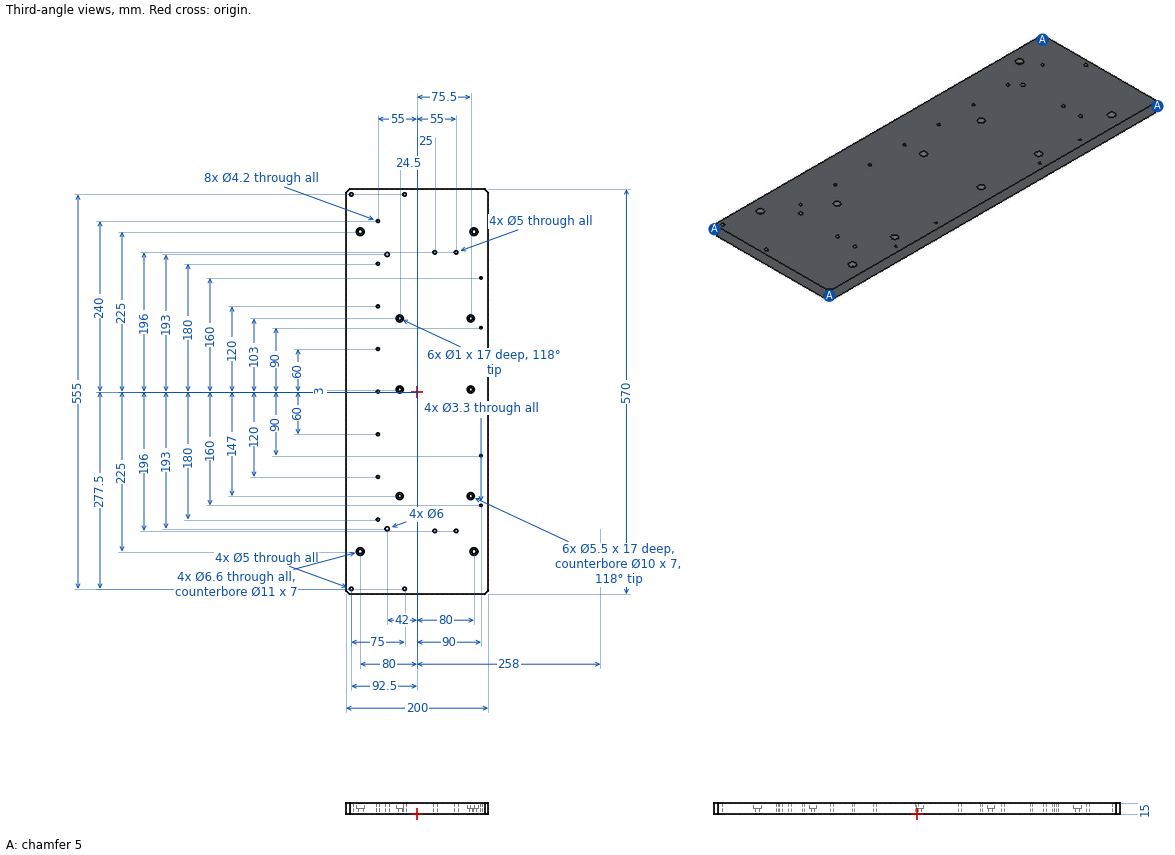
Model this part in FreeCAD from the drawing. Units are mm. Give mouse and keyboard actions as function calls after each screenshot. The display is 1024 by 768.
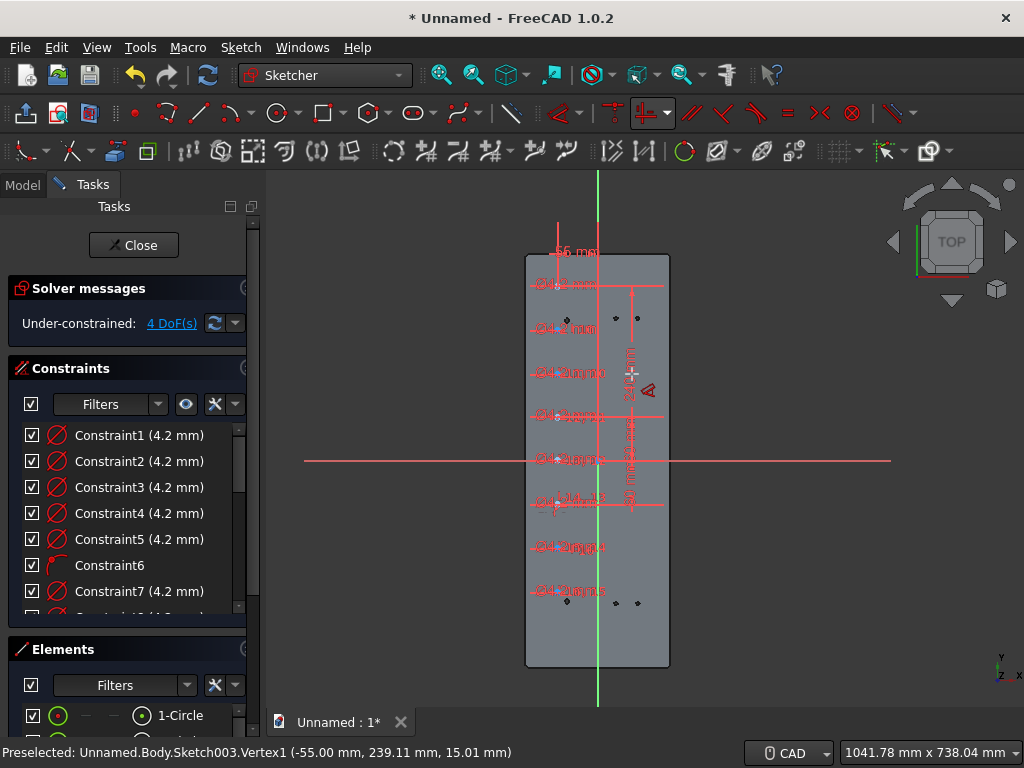
click(558, 331)
click(632, 396)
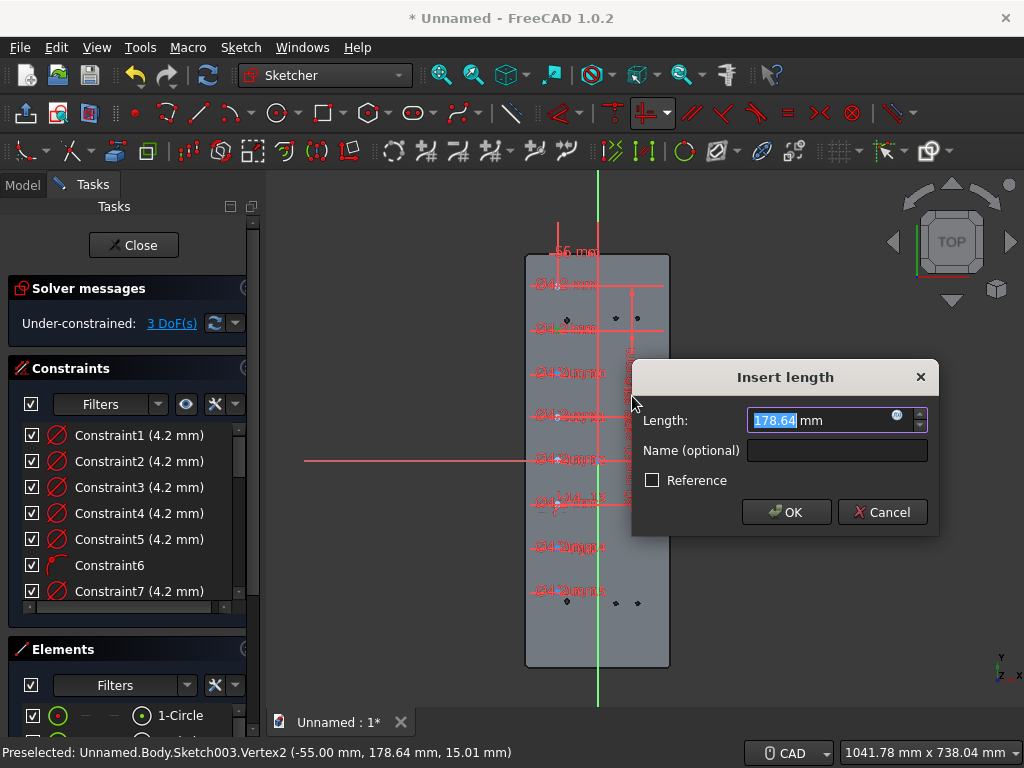
text(180)
key(Return)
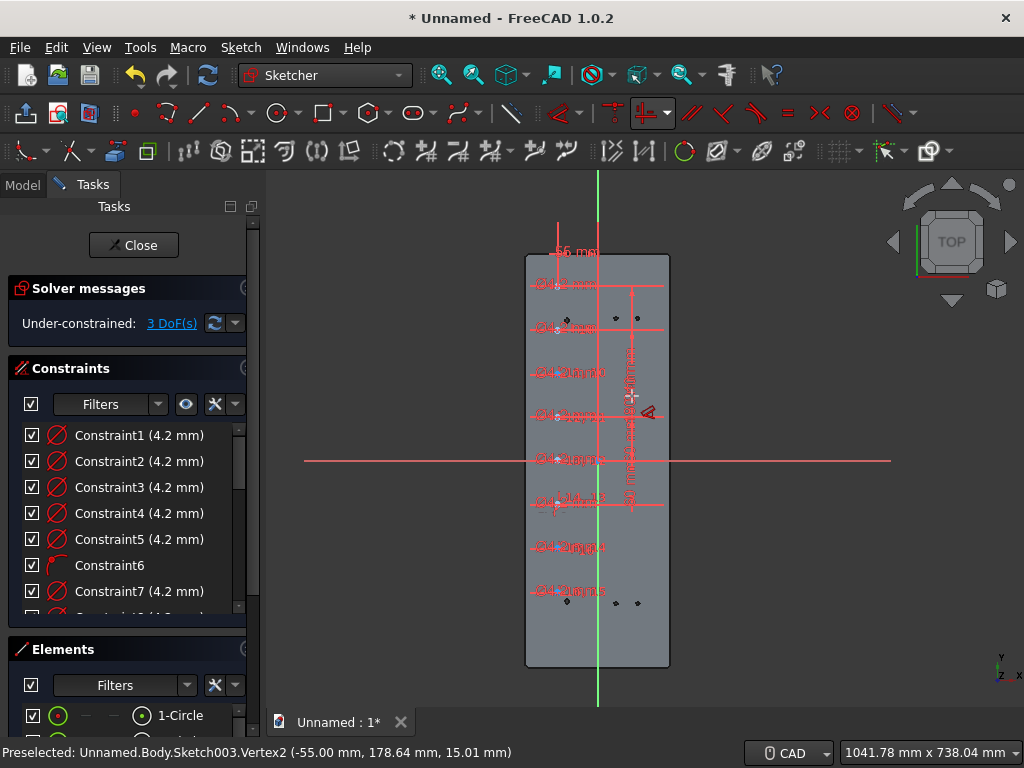
click(558, 375)
click(632, 418)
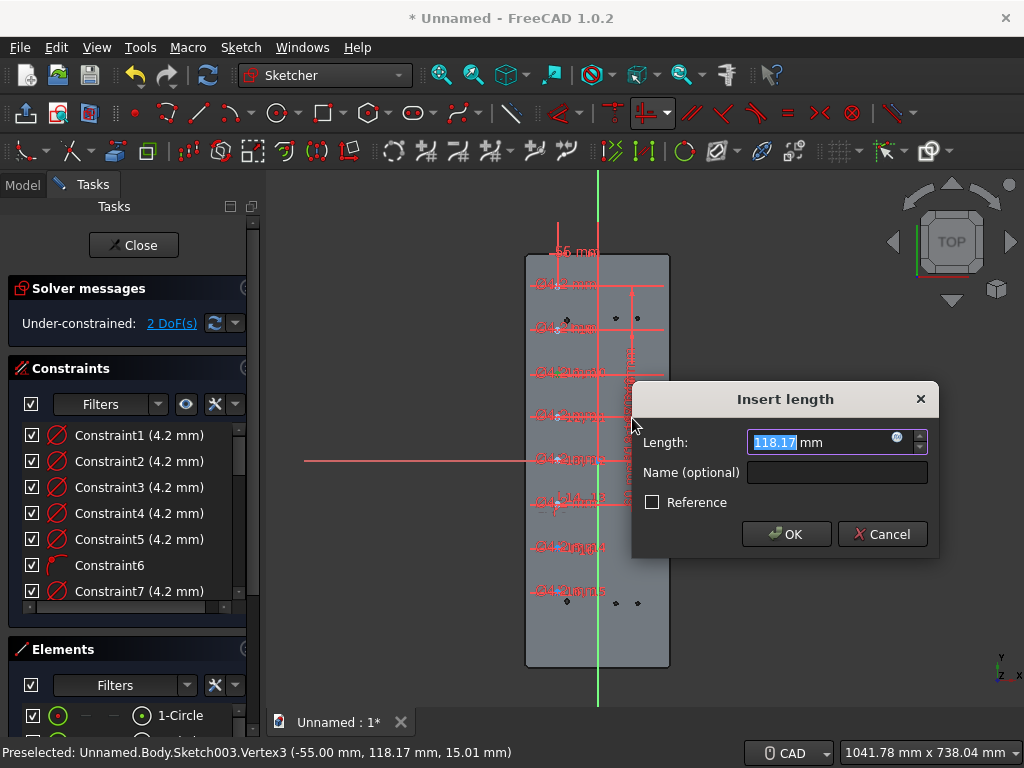
text(120)
key(Return)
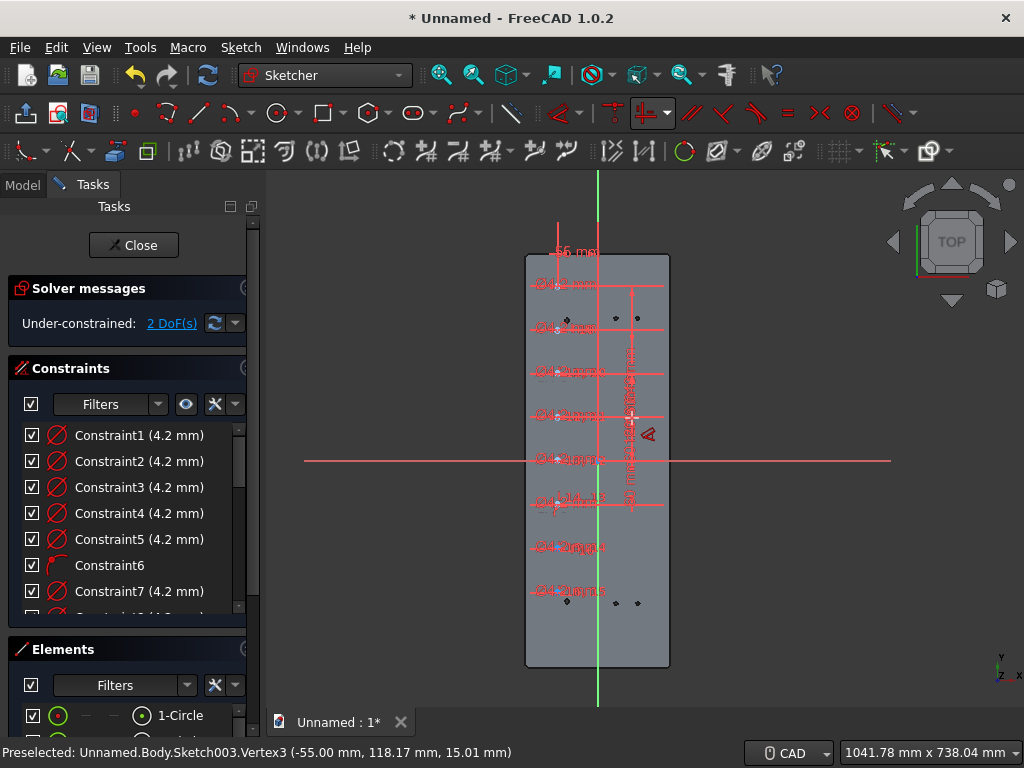
click(558, 549)
click(632, 505)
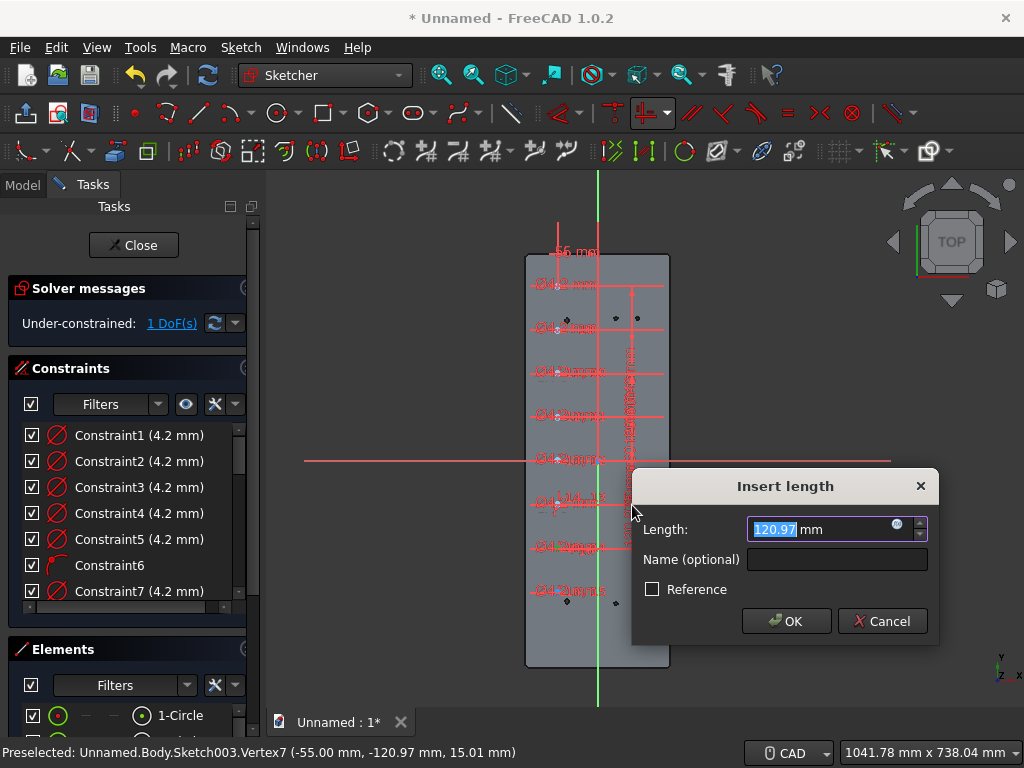
text(120)
key(Return)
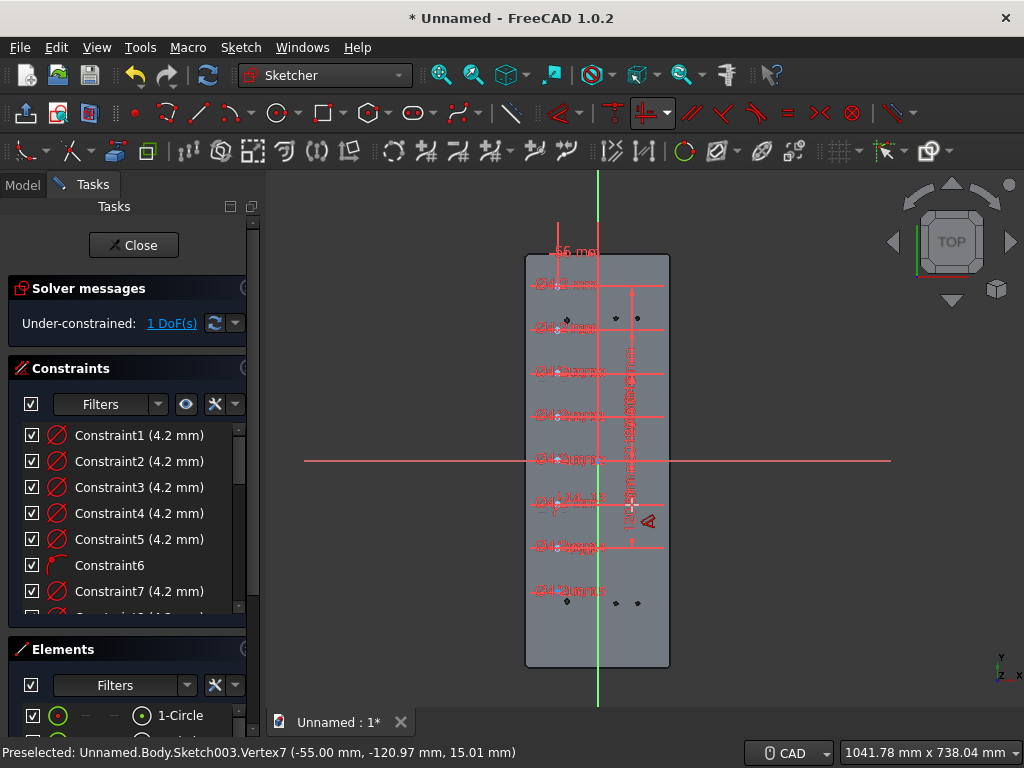
click(558, 593)
click(632, 527)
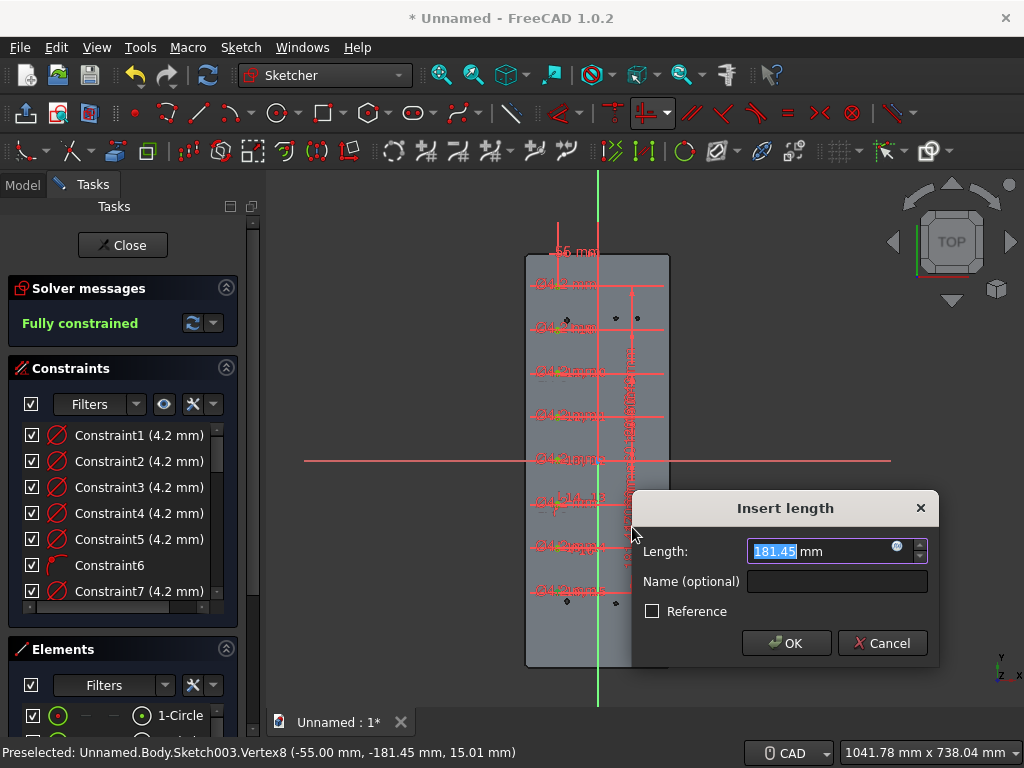
text(180)
key(Return)
key(Escape)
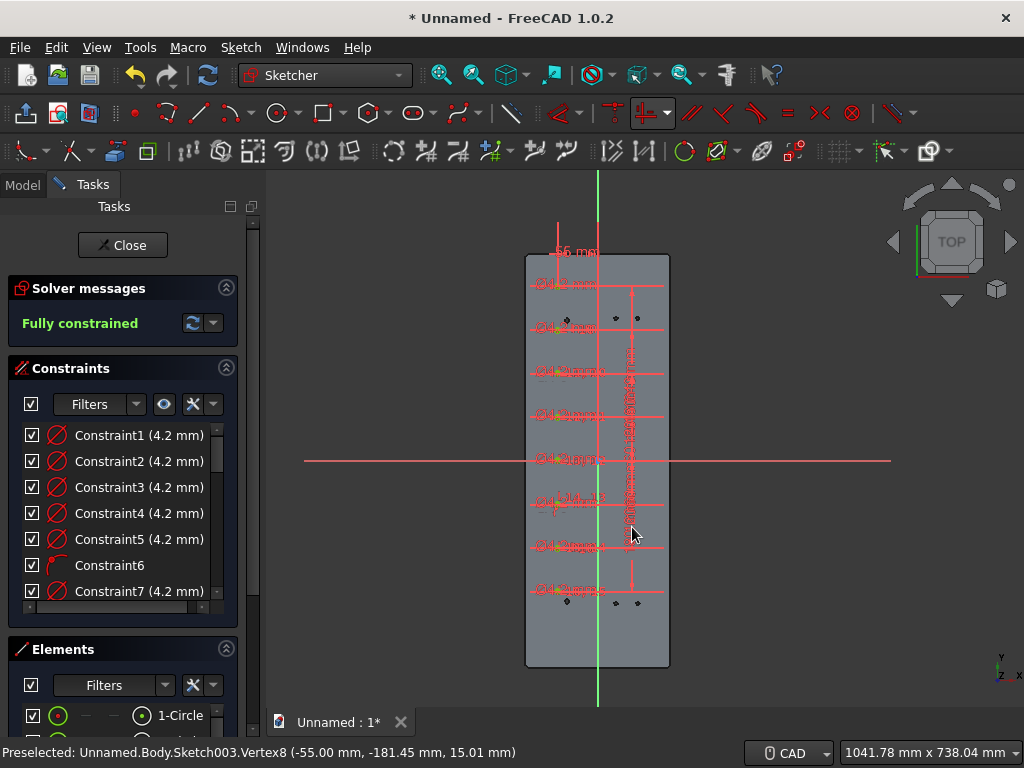
click(123, 245)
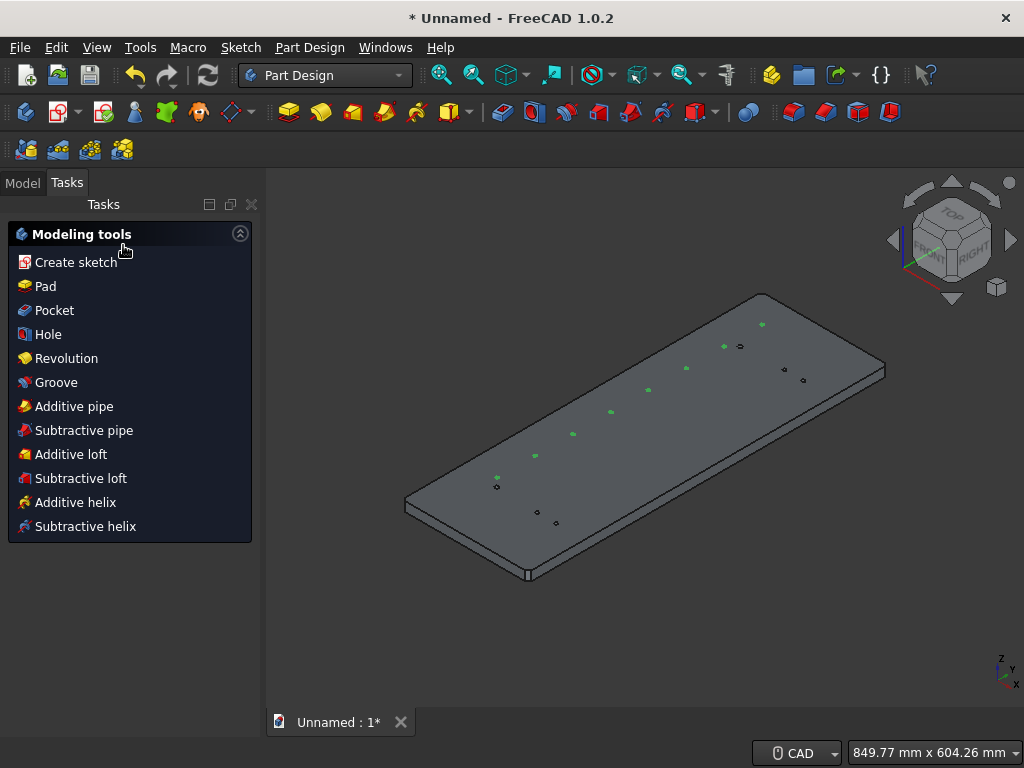
click(536, 112)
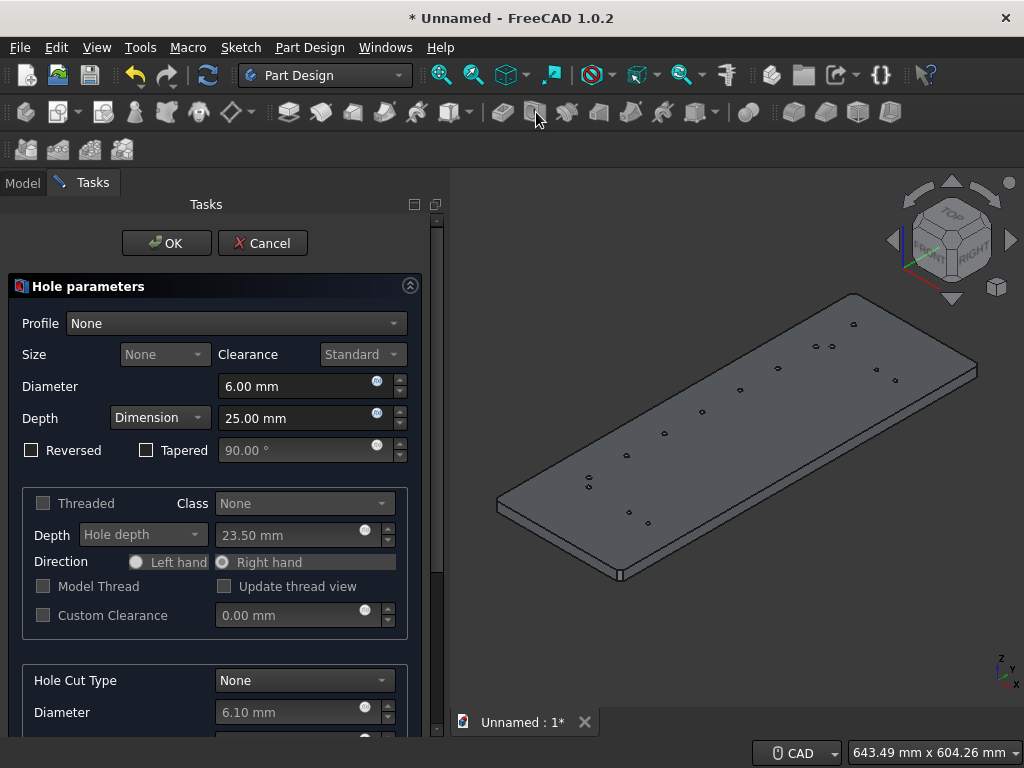
triple_click(305, 386)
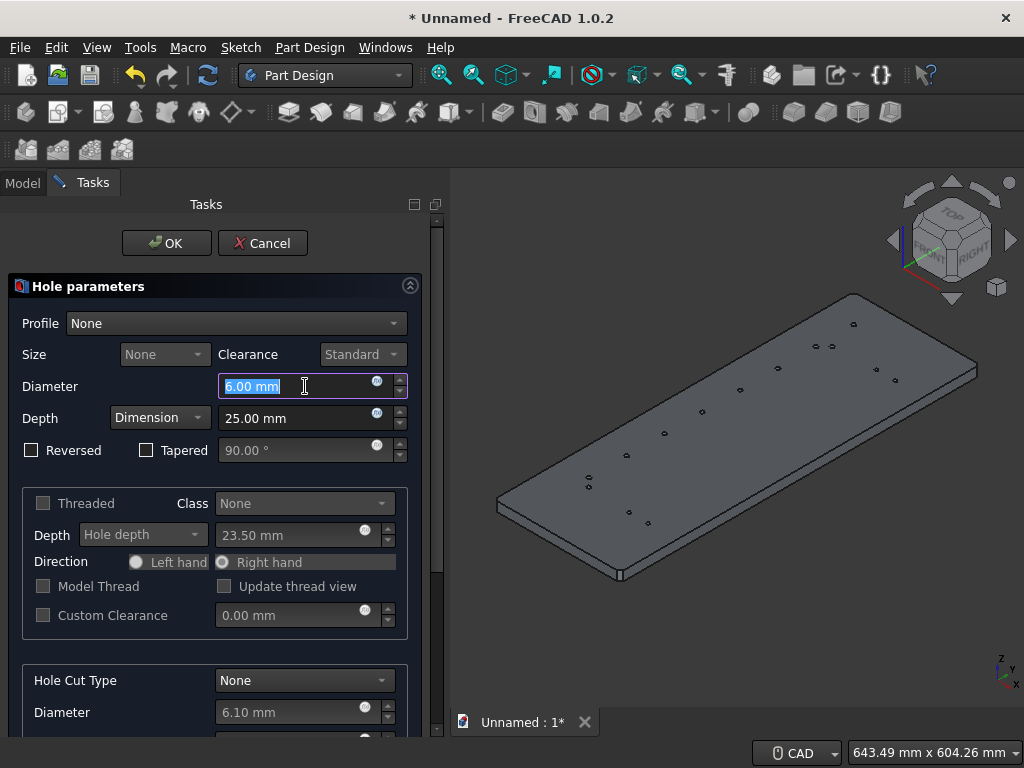
text(4.2)
key(Tab)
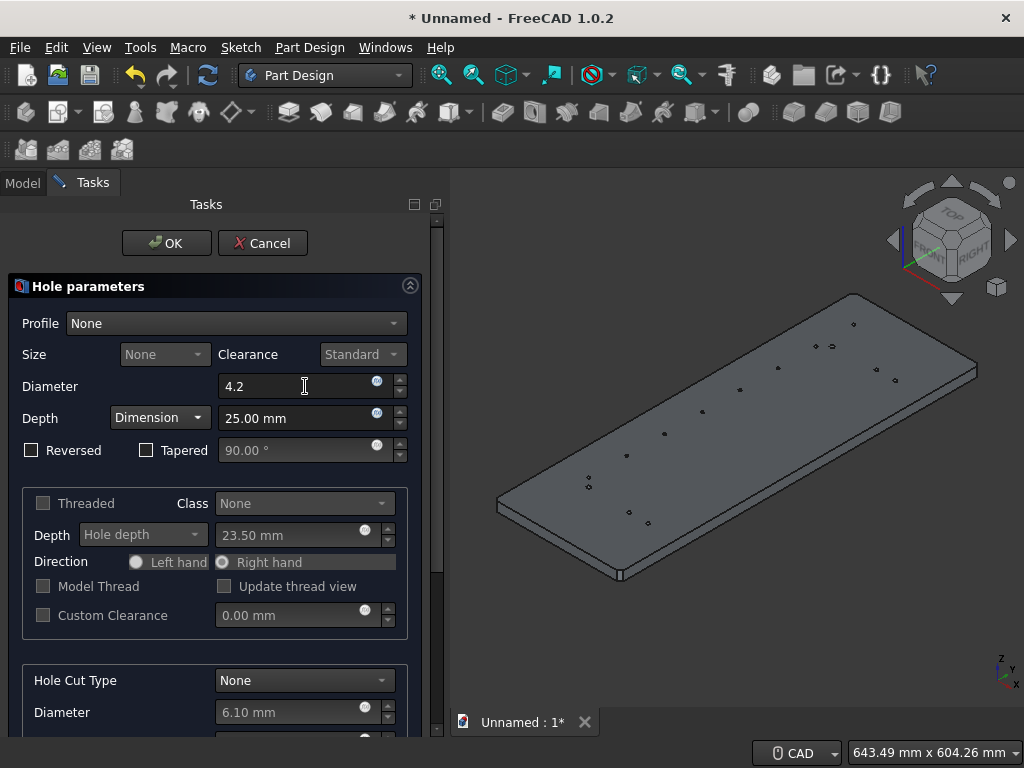
click(161, 418)